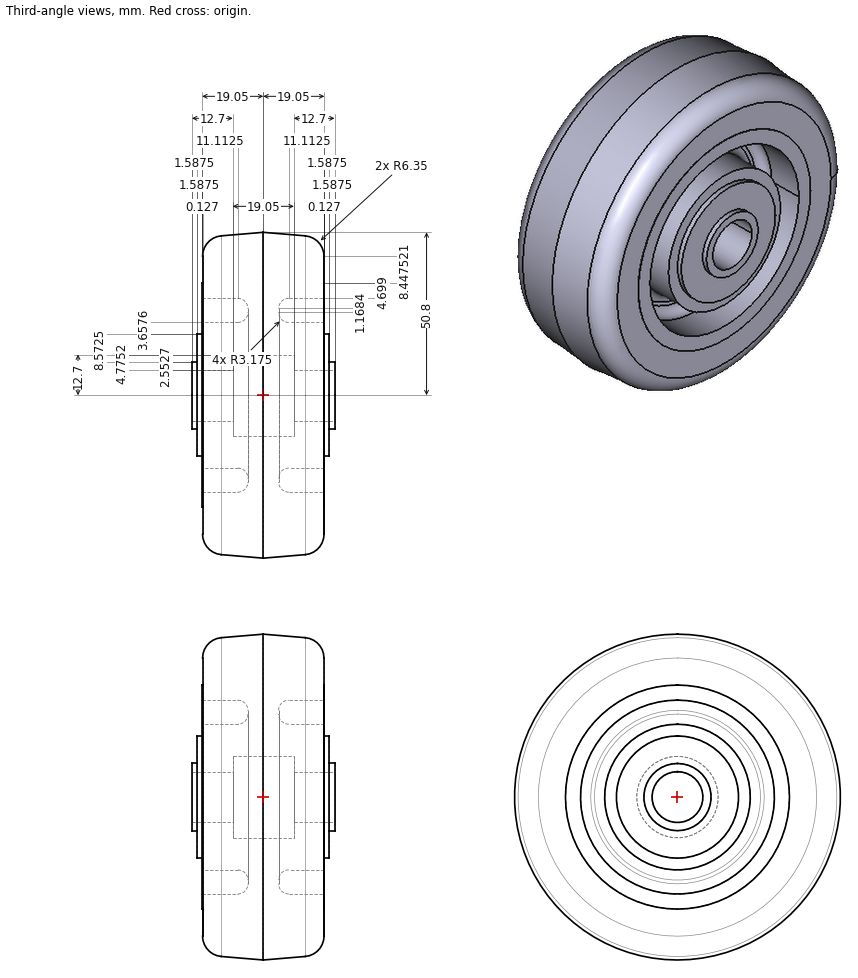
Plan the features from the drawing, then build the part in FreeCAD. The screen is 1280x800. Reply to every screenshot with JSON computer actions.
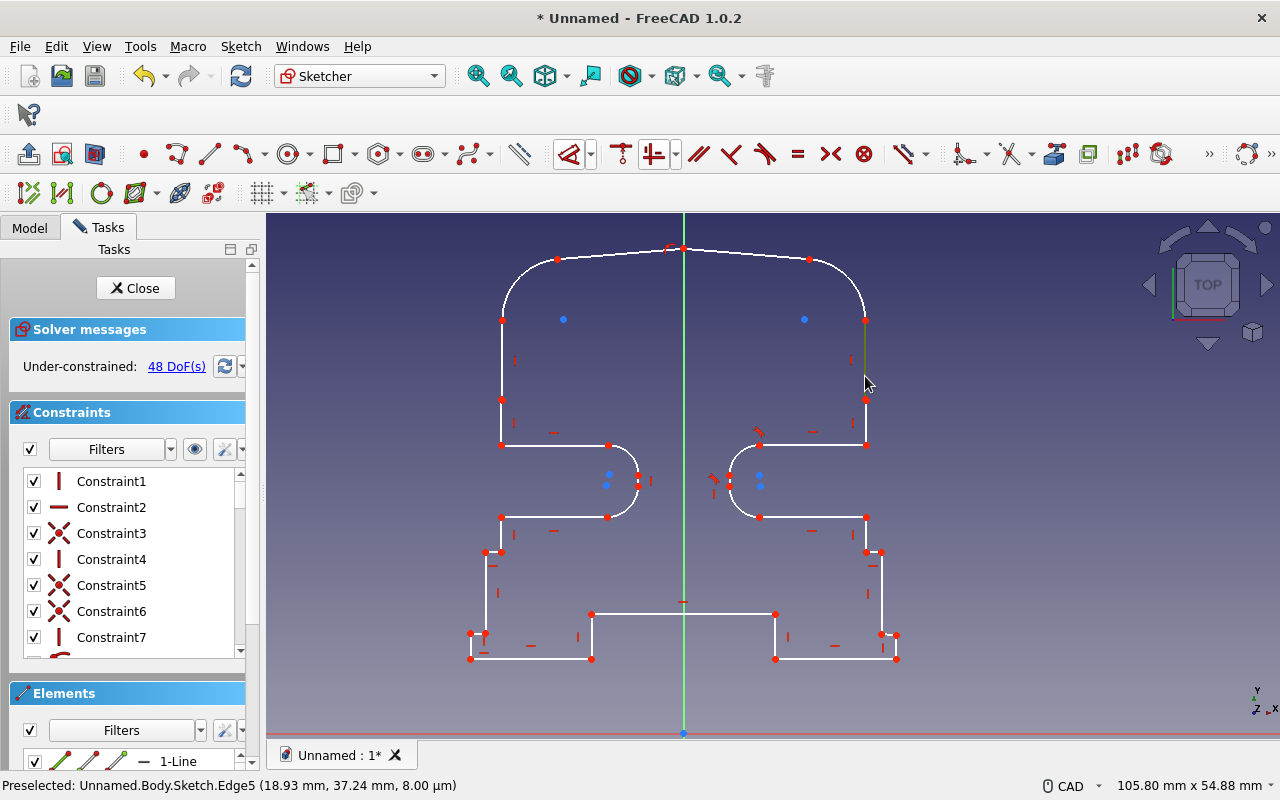
{"action": "left_click", "coordinate": [859, 294]}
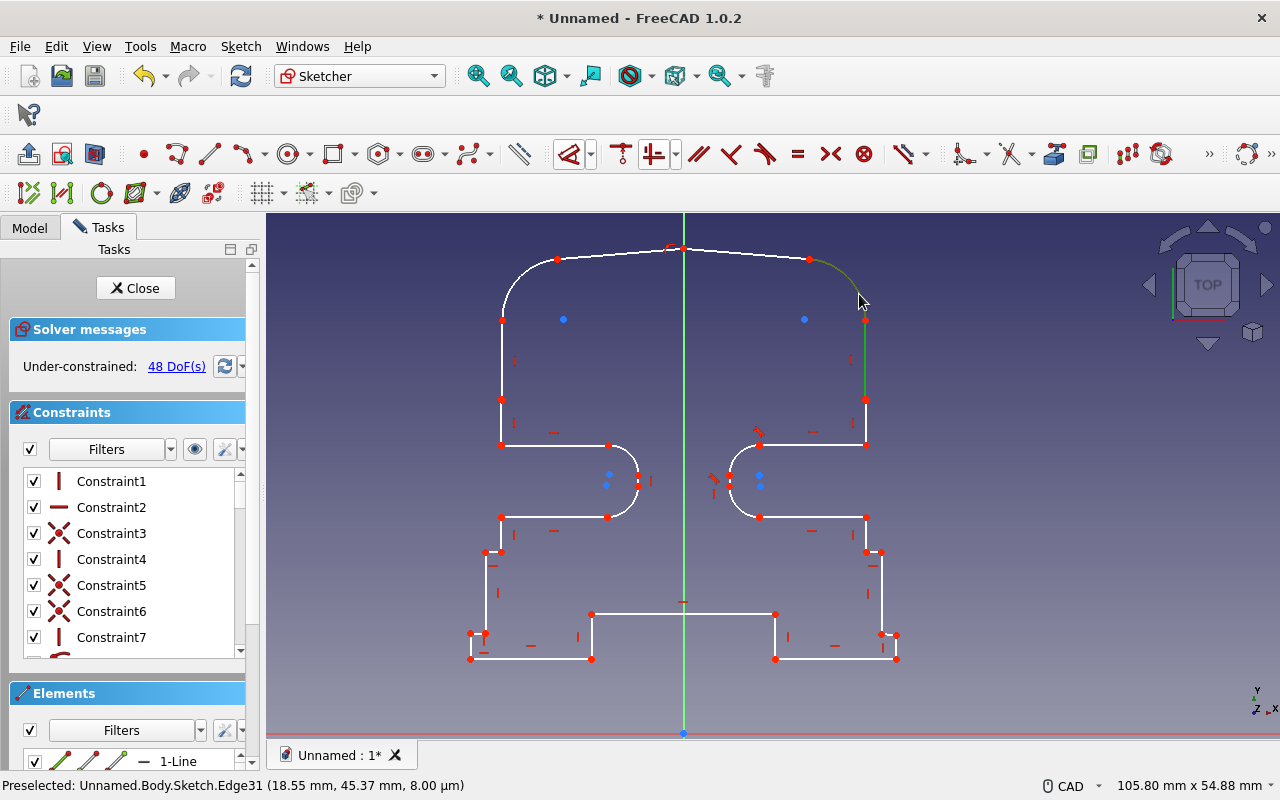
{"action": "left_click", "coordinate": [765, 154]}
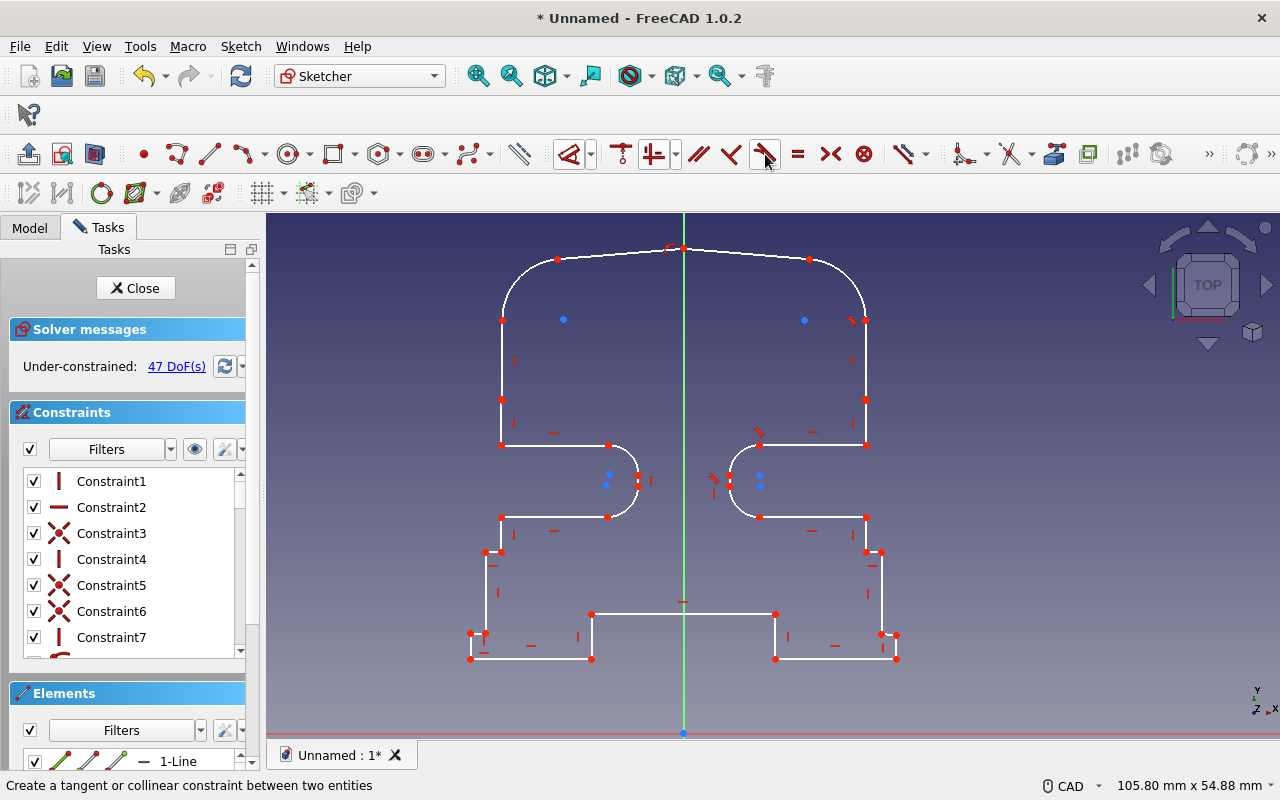
{"action": "left_click", "coordinate": [772, 256]}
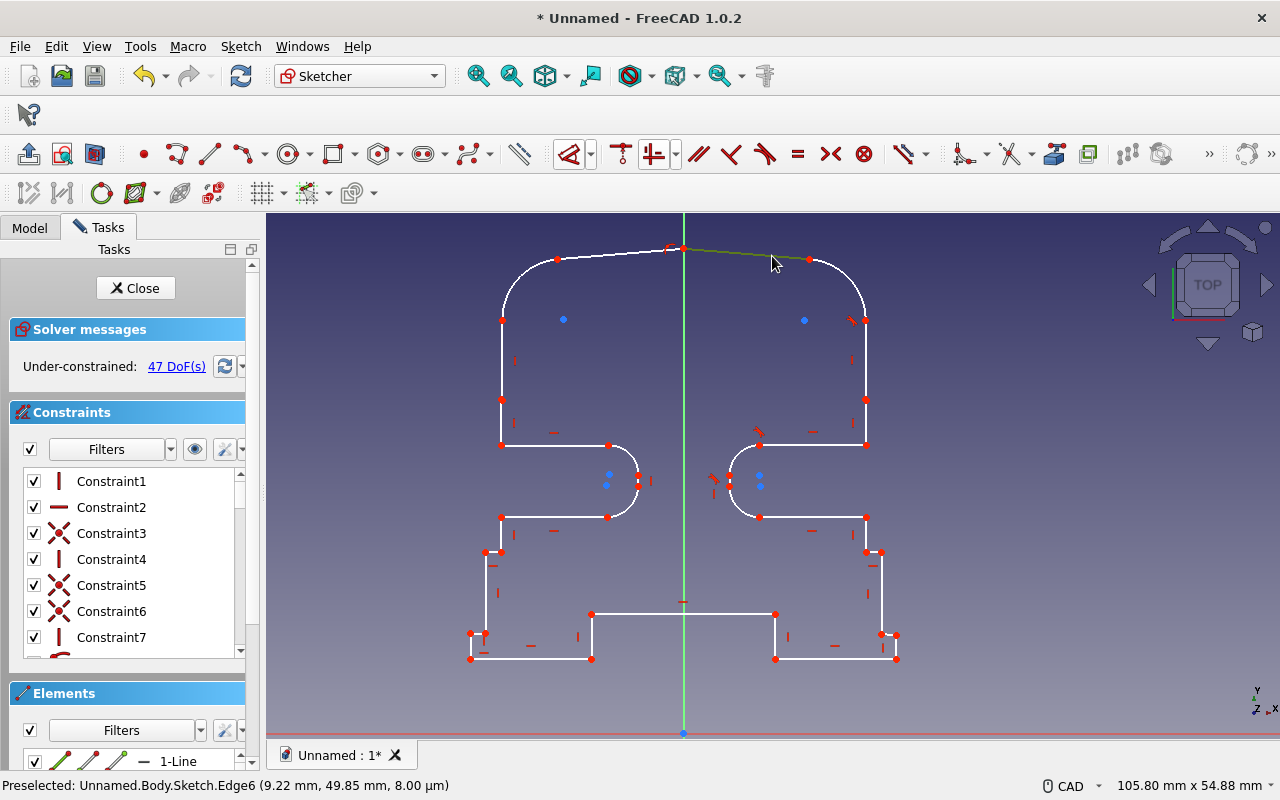
{"action": "left_click", "coordinate": [860, 294]}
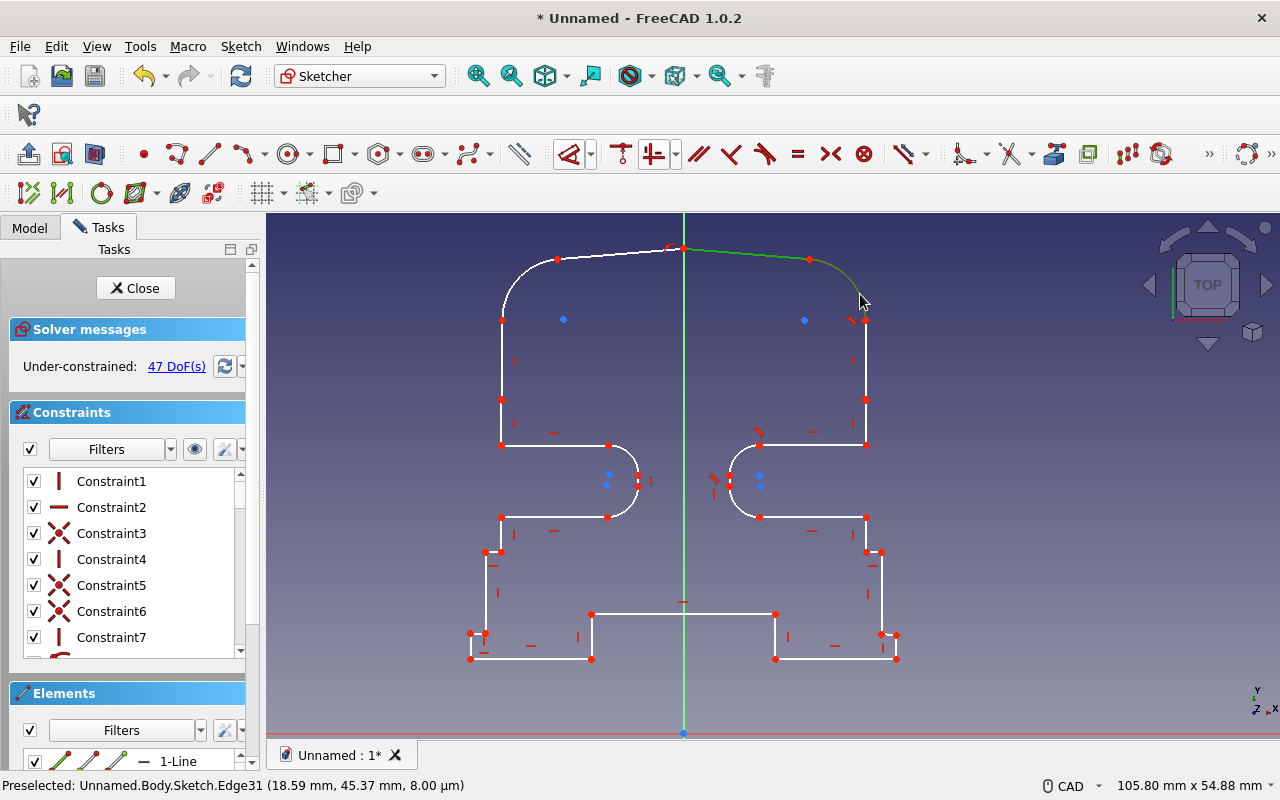
{"action": "left_click", "coordinate": [765, 154]}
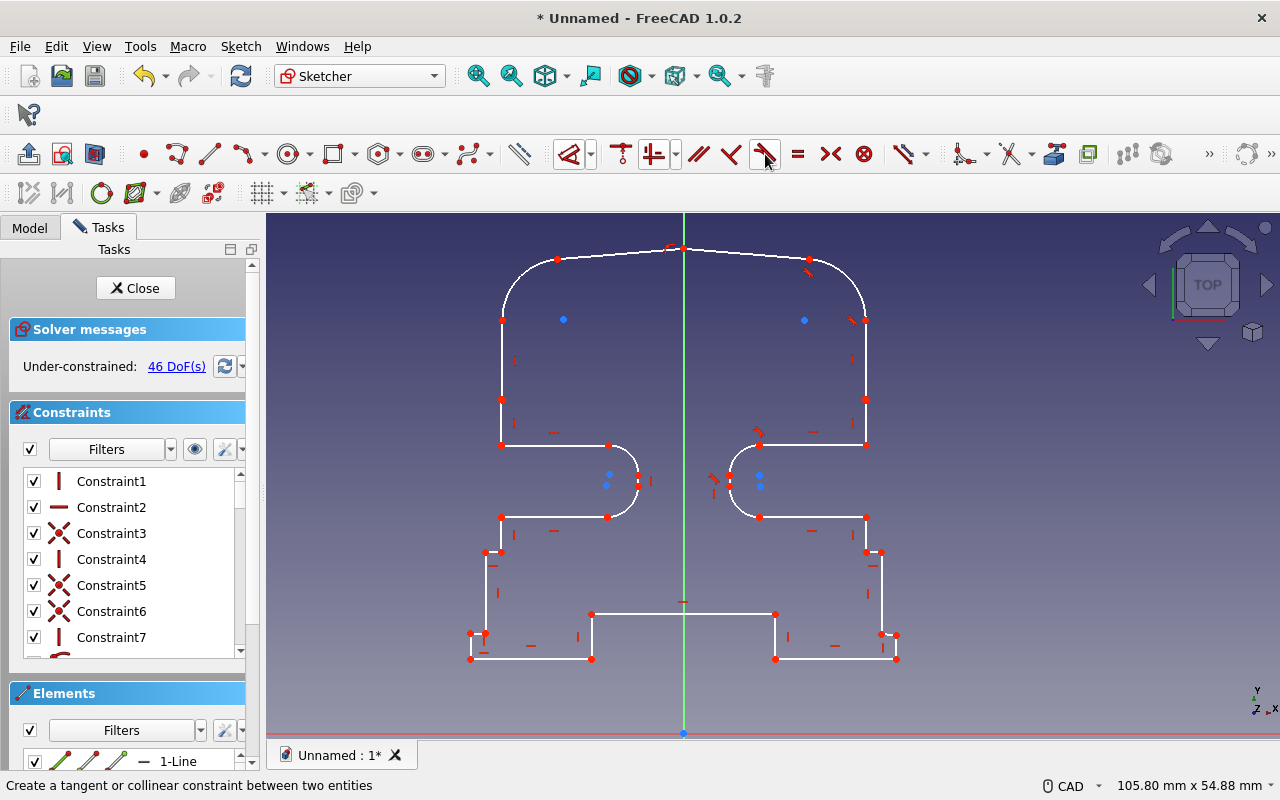
{"action": "left_click", "coordinate": [646, 252]}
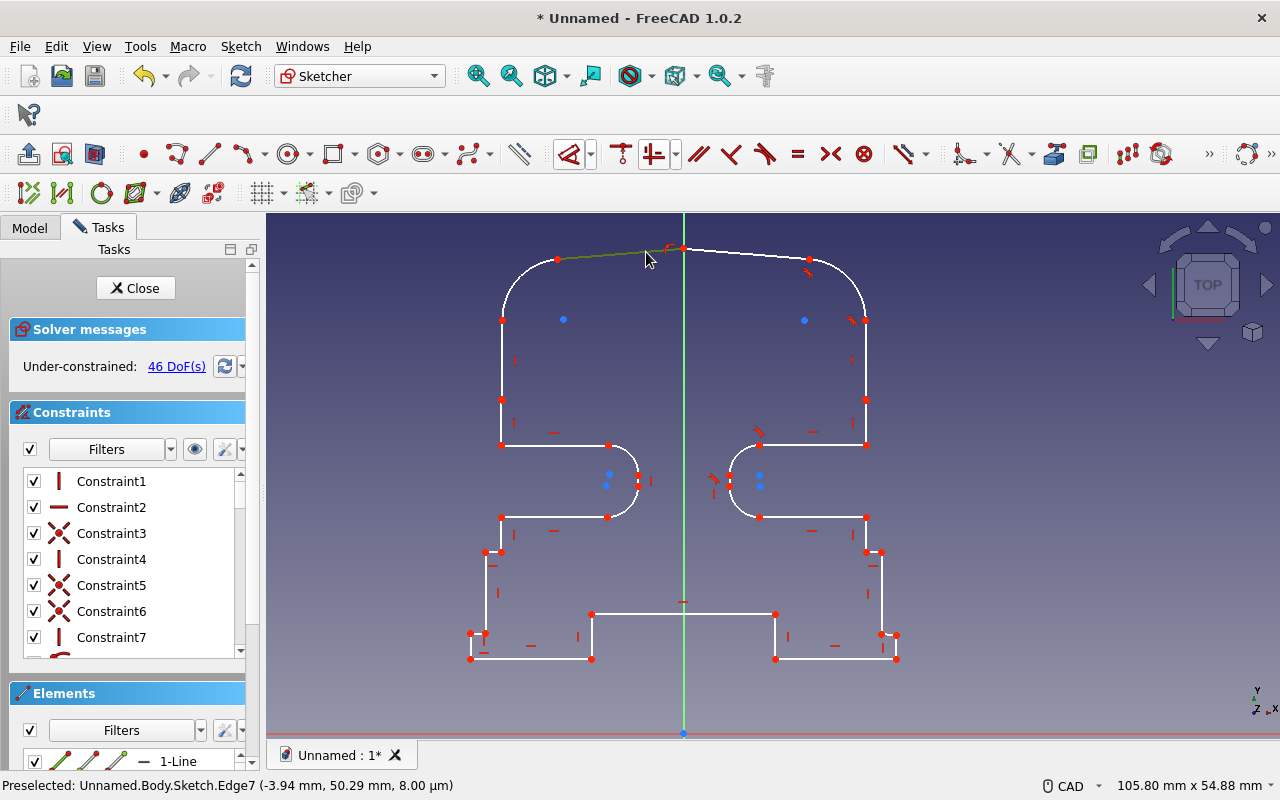
{"action": "left_click", "coordinate": [532, 268]}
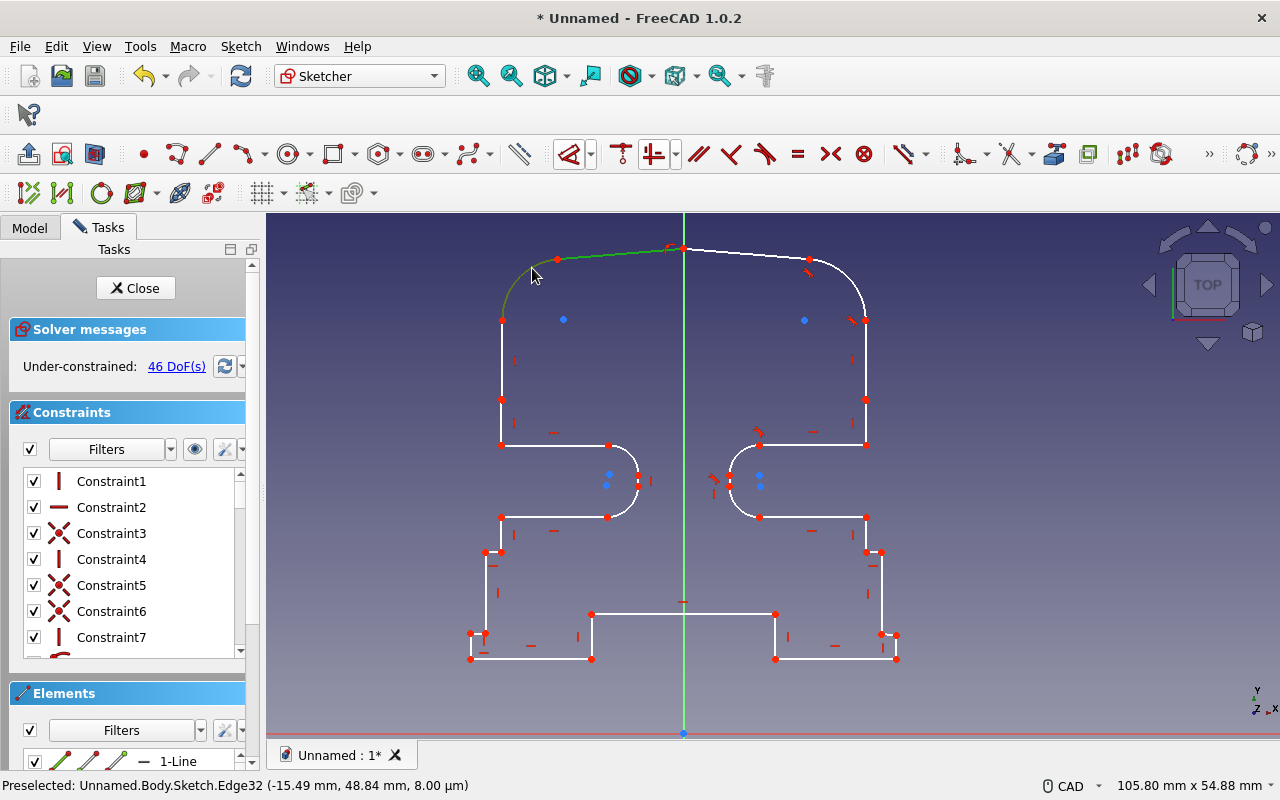
{"action": "left_click", "coordinate": [765, 154]}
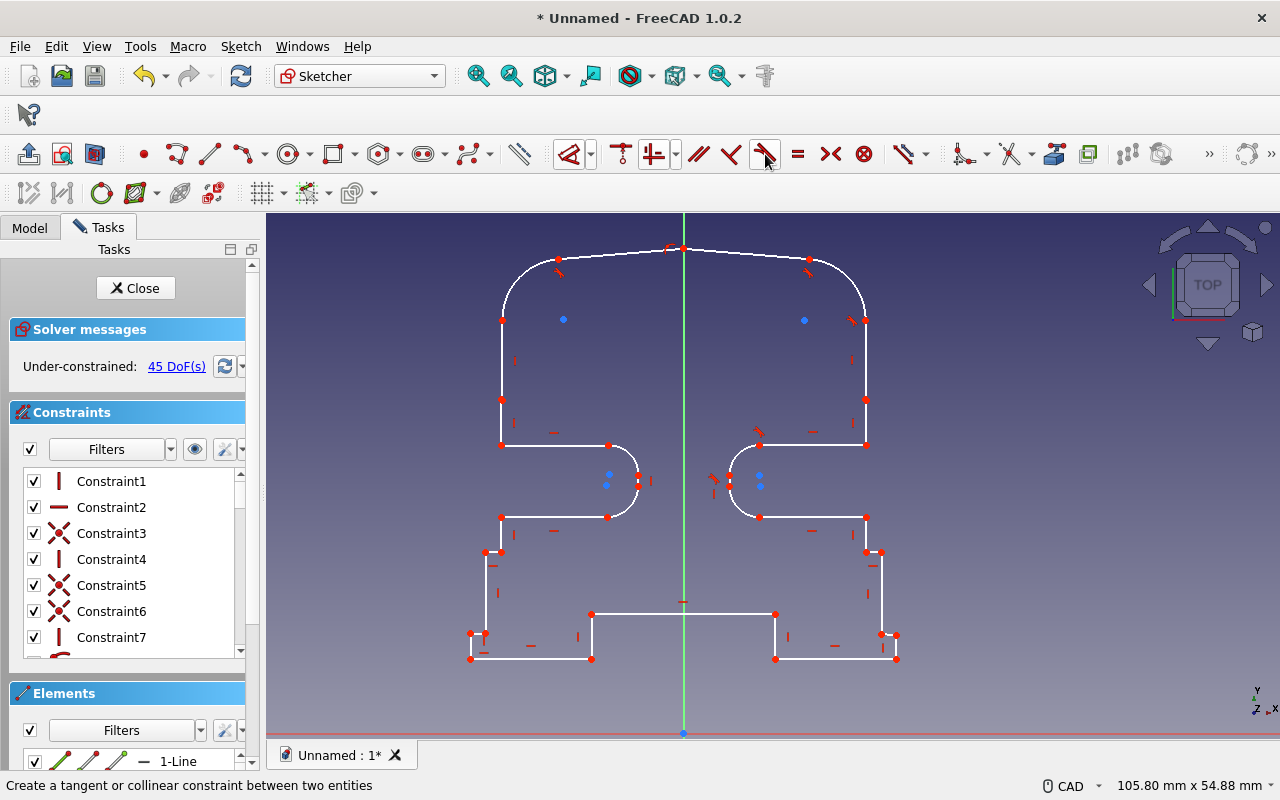
{"action": "left_click", "coordinate": [502, 345]}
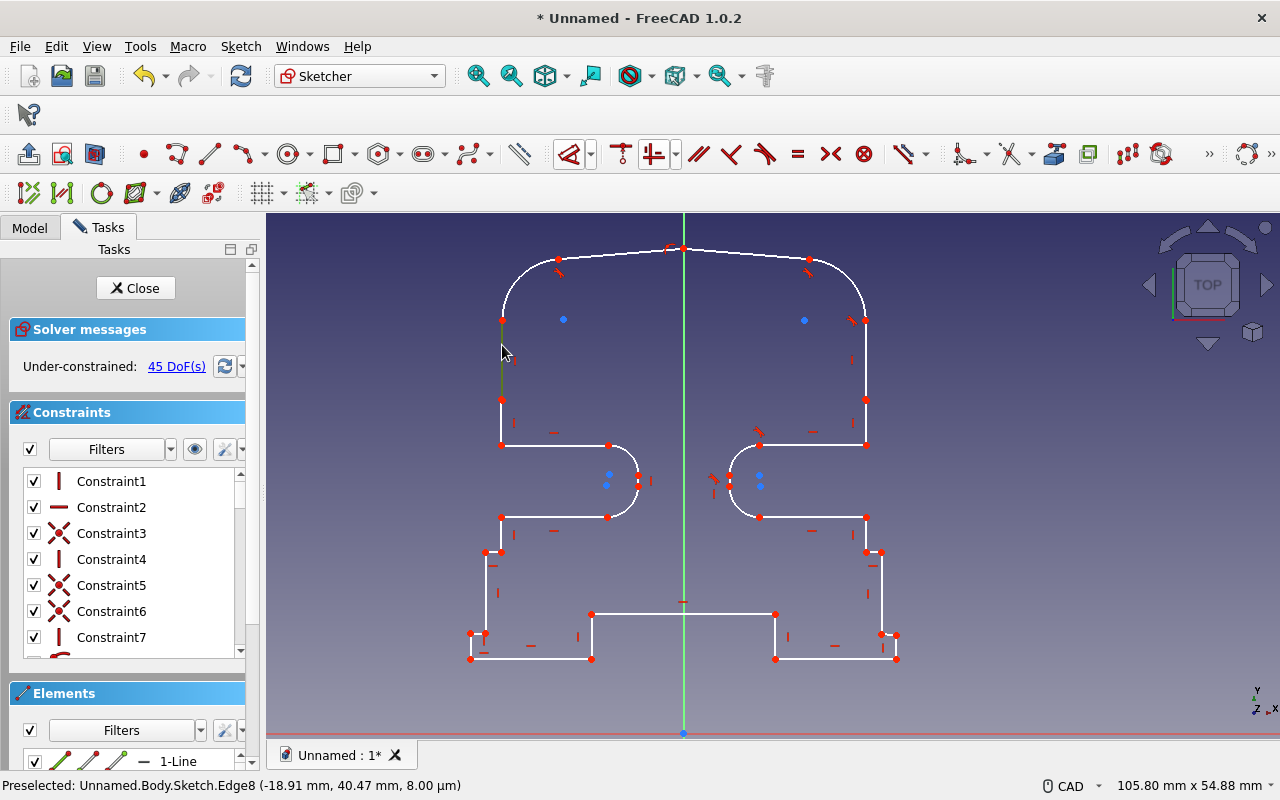
{"action": "left_click", "coordinate": [532, 267]}